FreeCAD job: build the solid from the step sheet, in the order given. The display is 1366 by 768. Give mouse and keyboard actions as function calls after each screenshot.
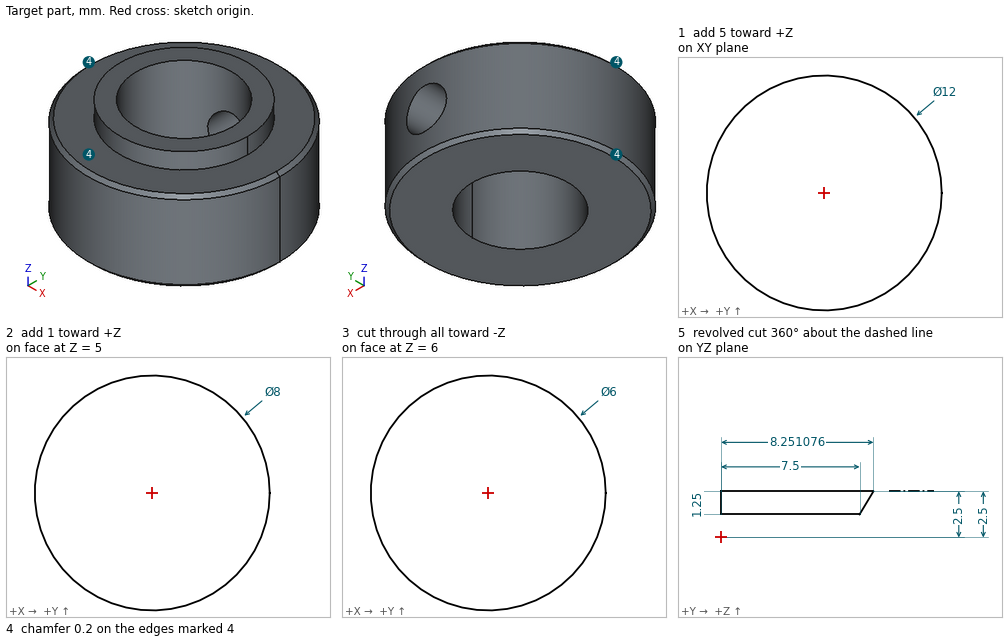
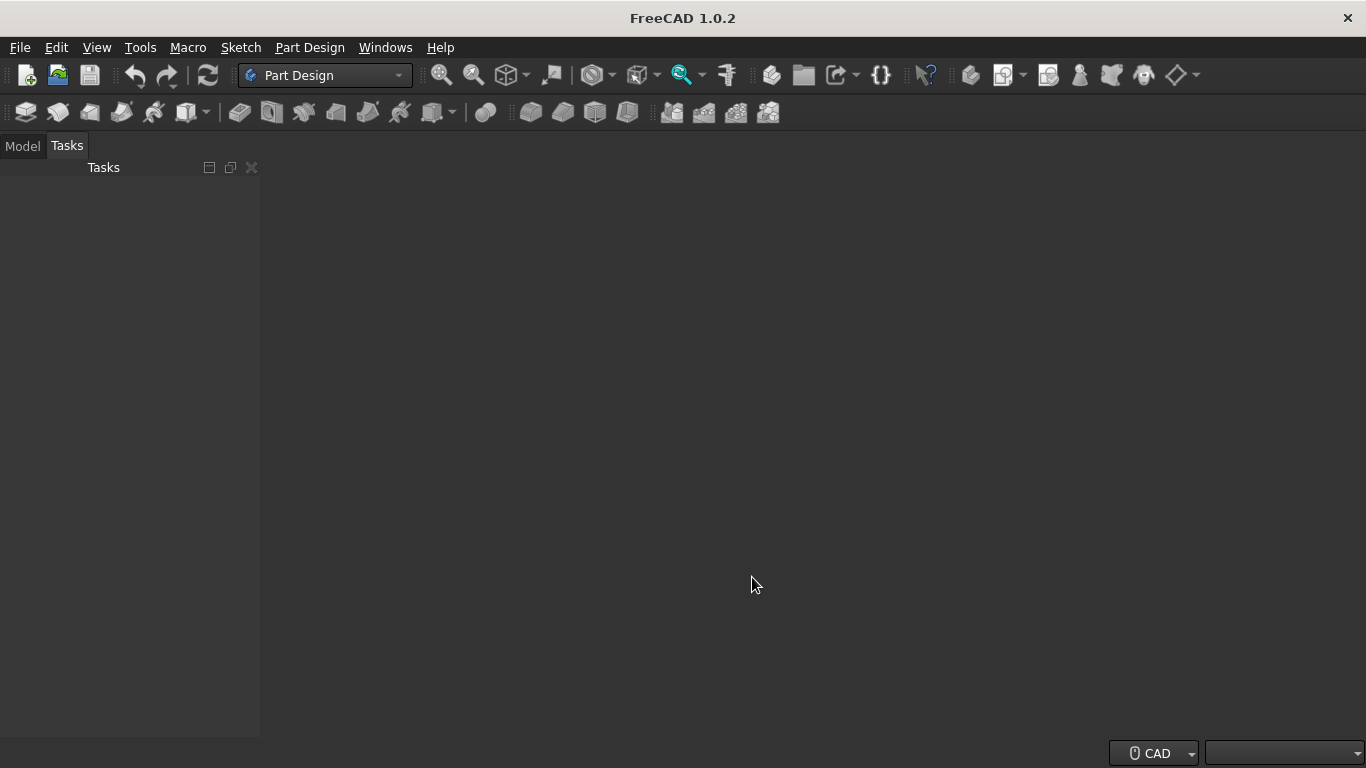
key(ctrl+n)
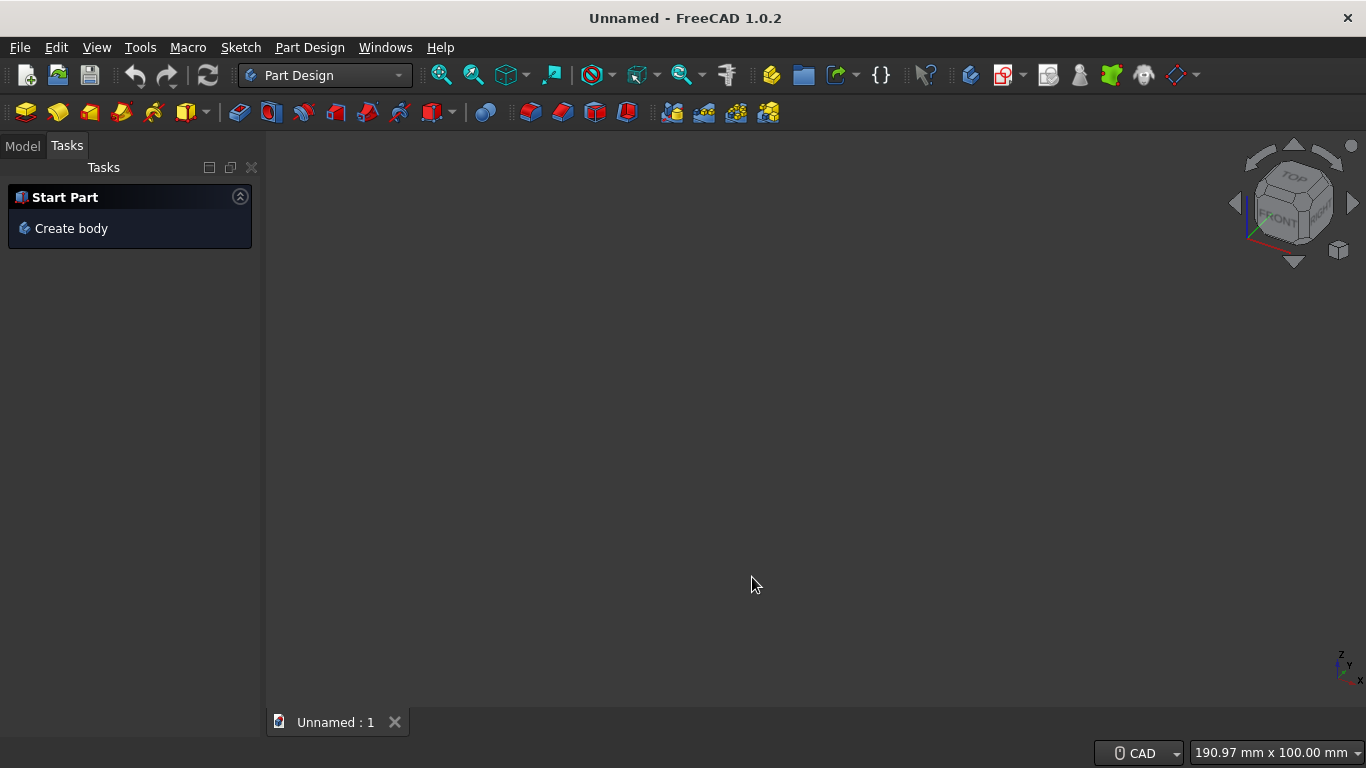
click(1004, 76)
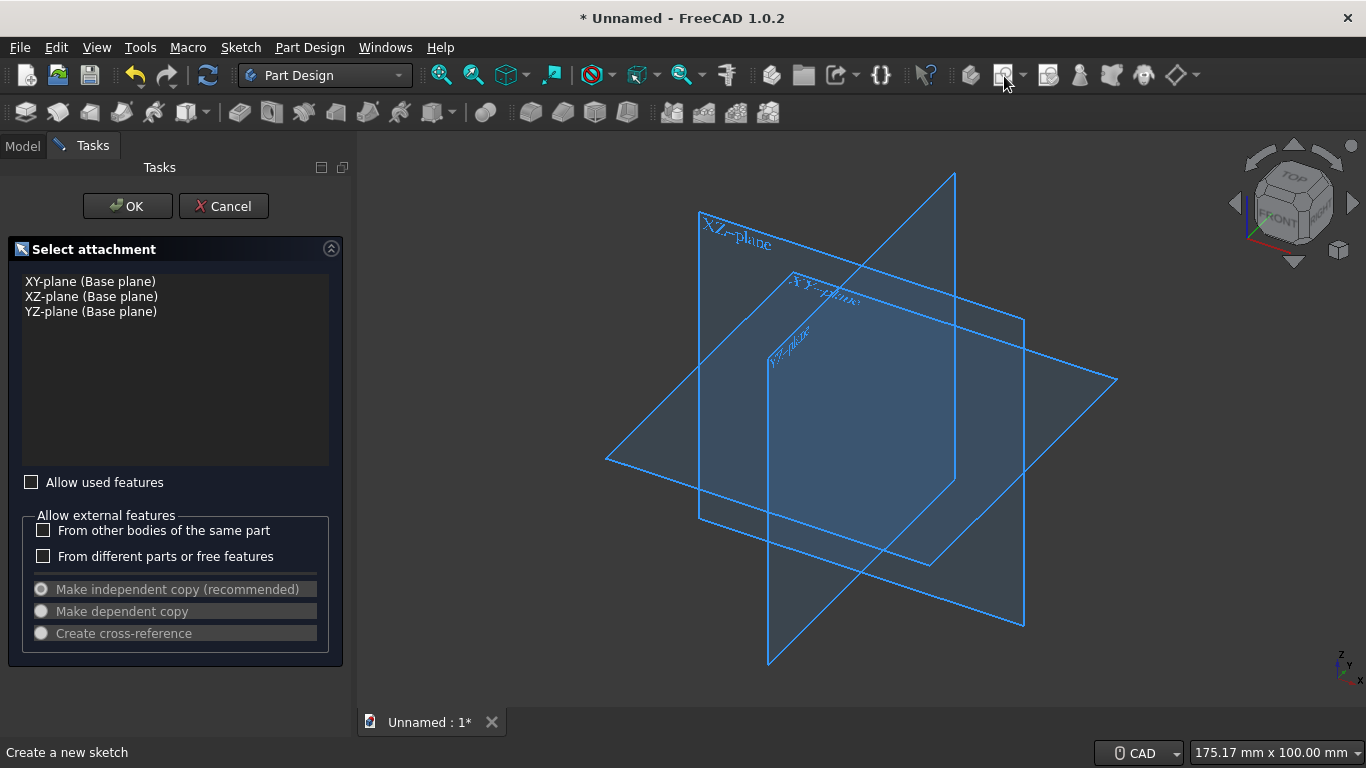
click(82, 282)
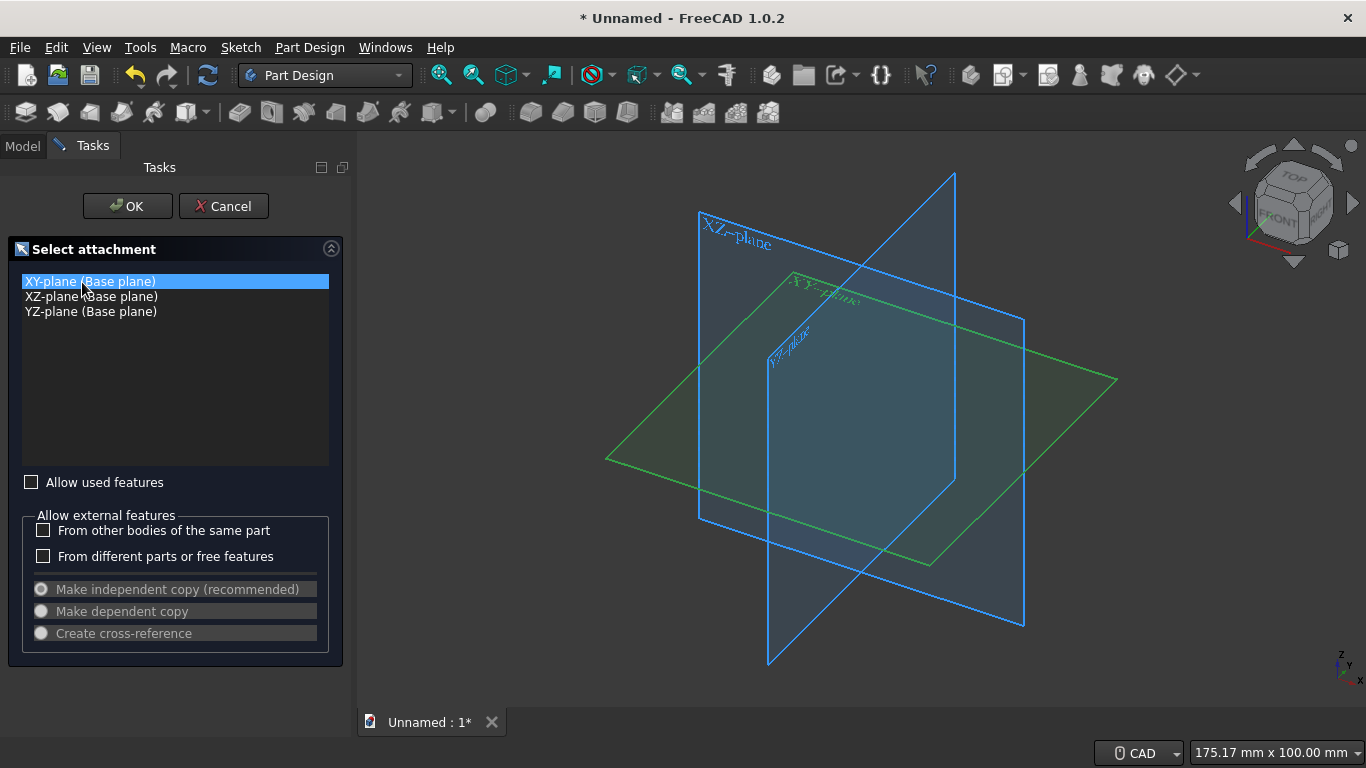
click(128, 206)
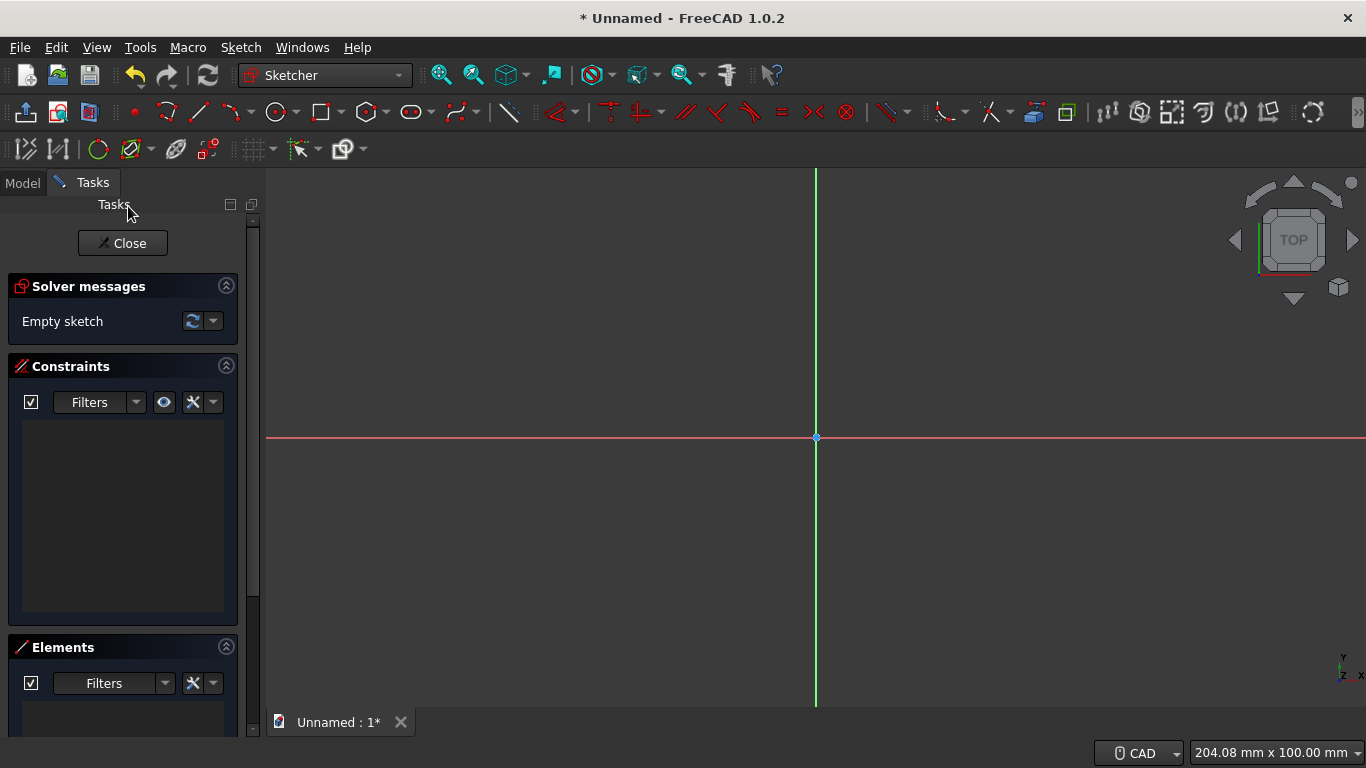
scroll(833, 438, up, 8)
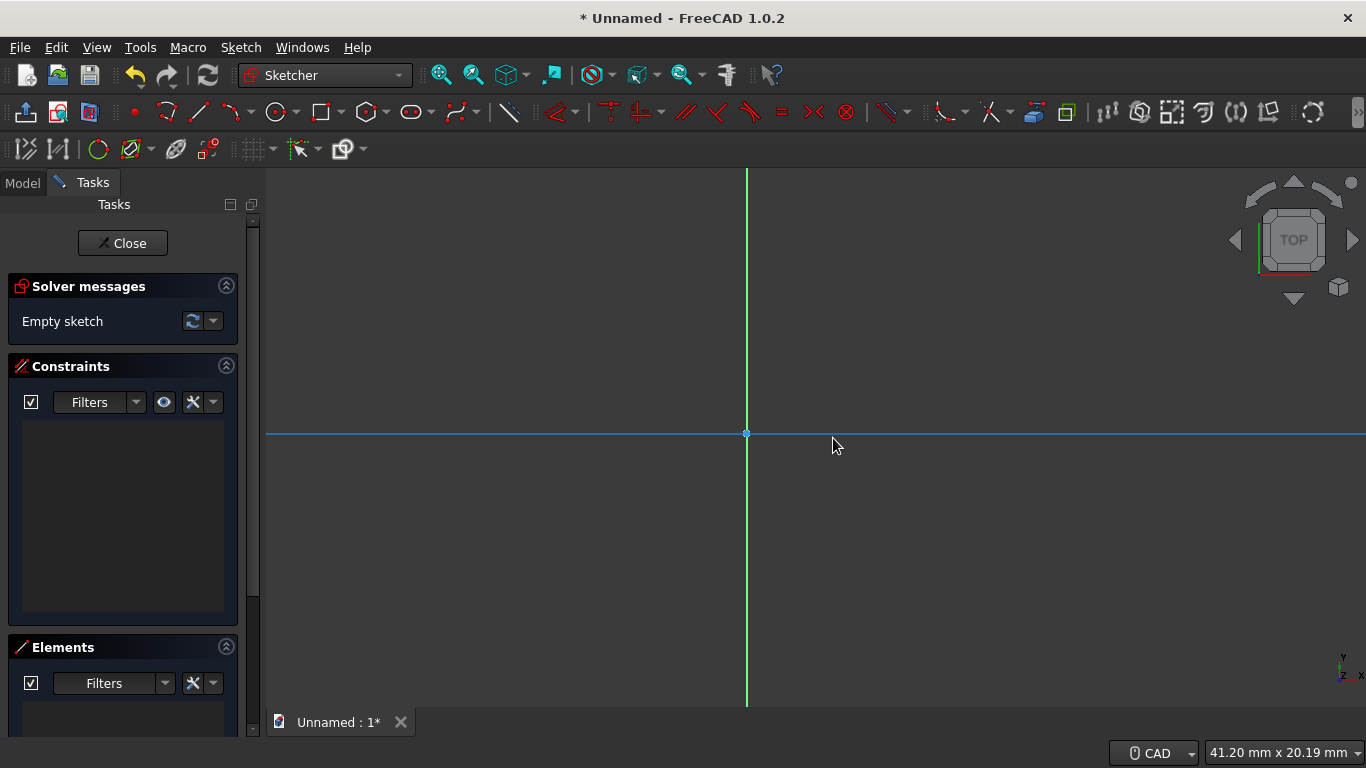
click(276, 112)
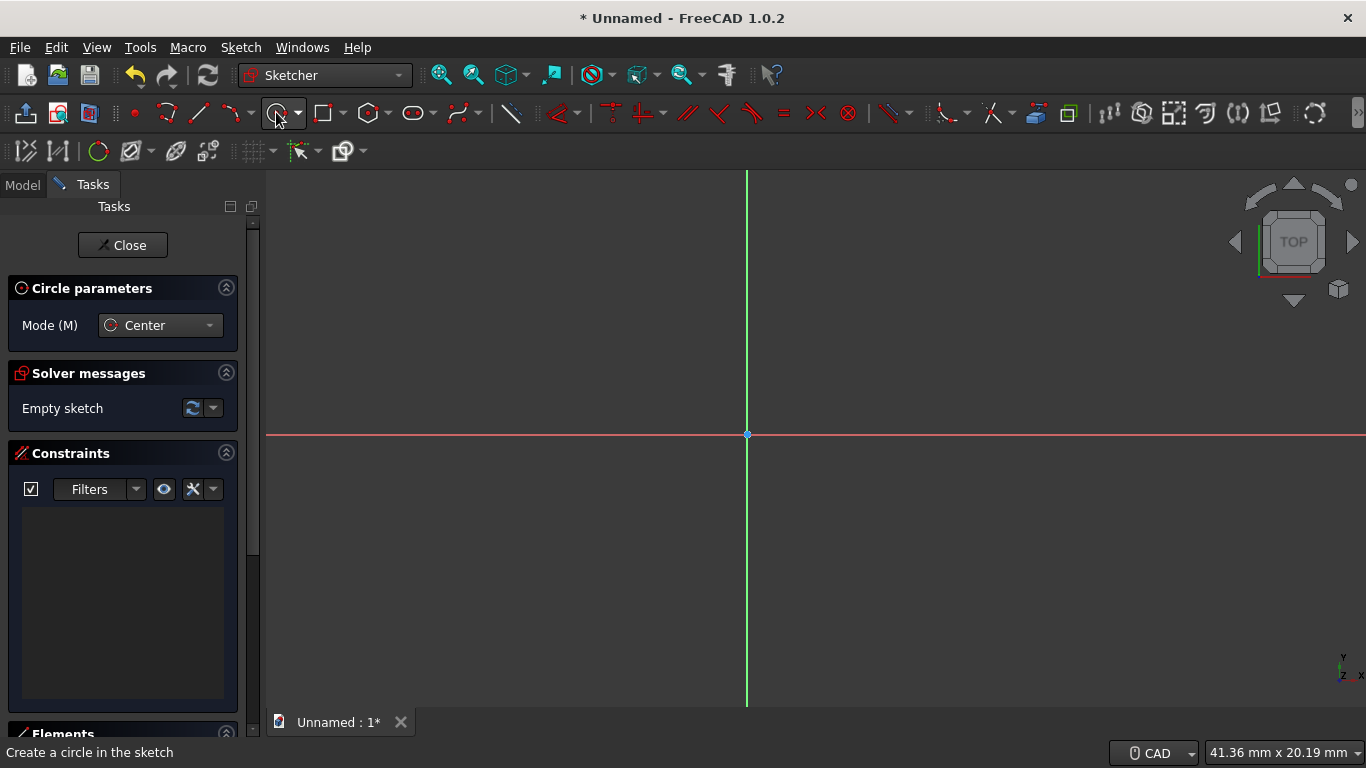
click(747, 435)
move(860, 322)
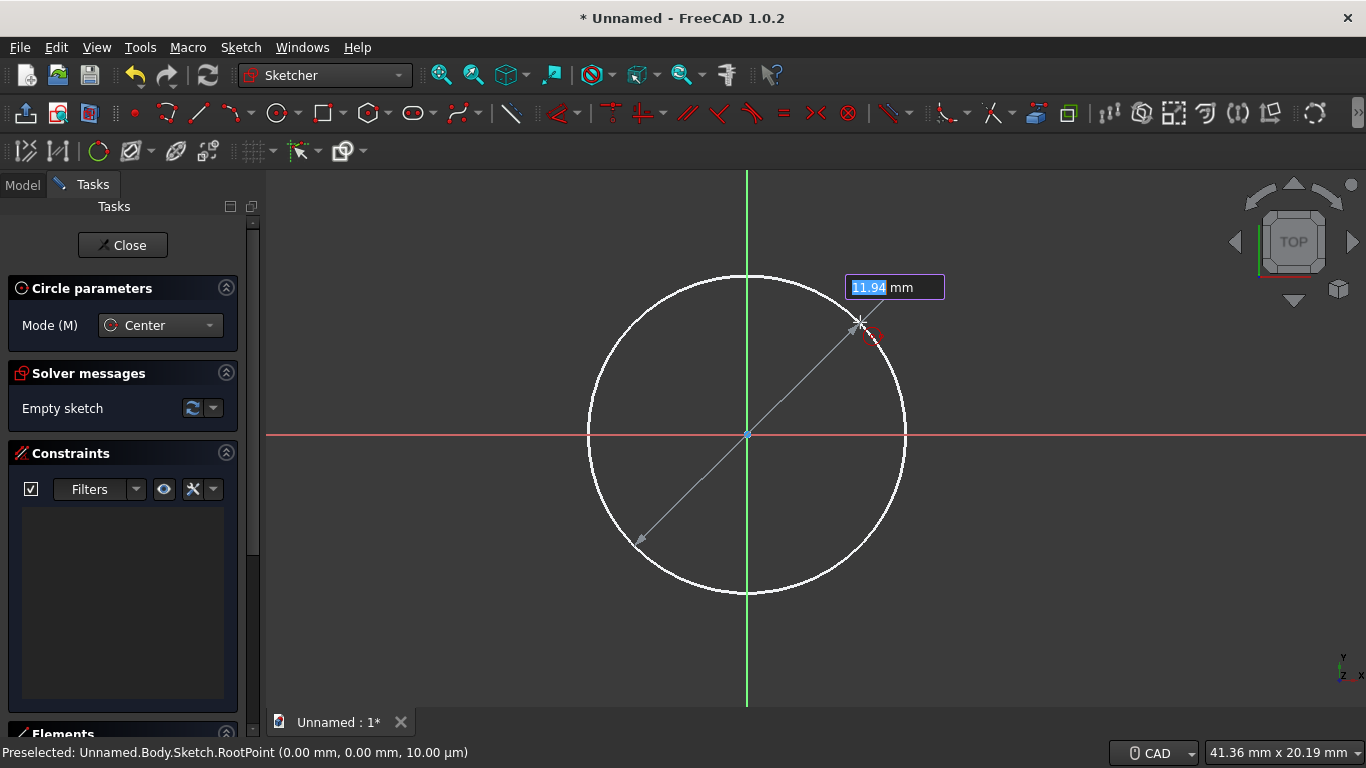
text(12)
key(Return)
key(Escape)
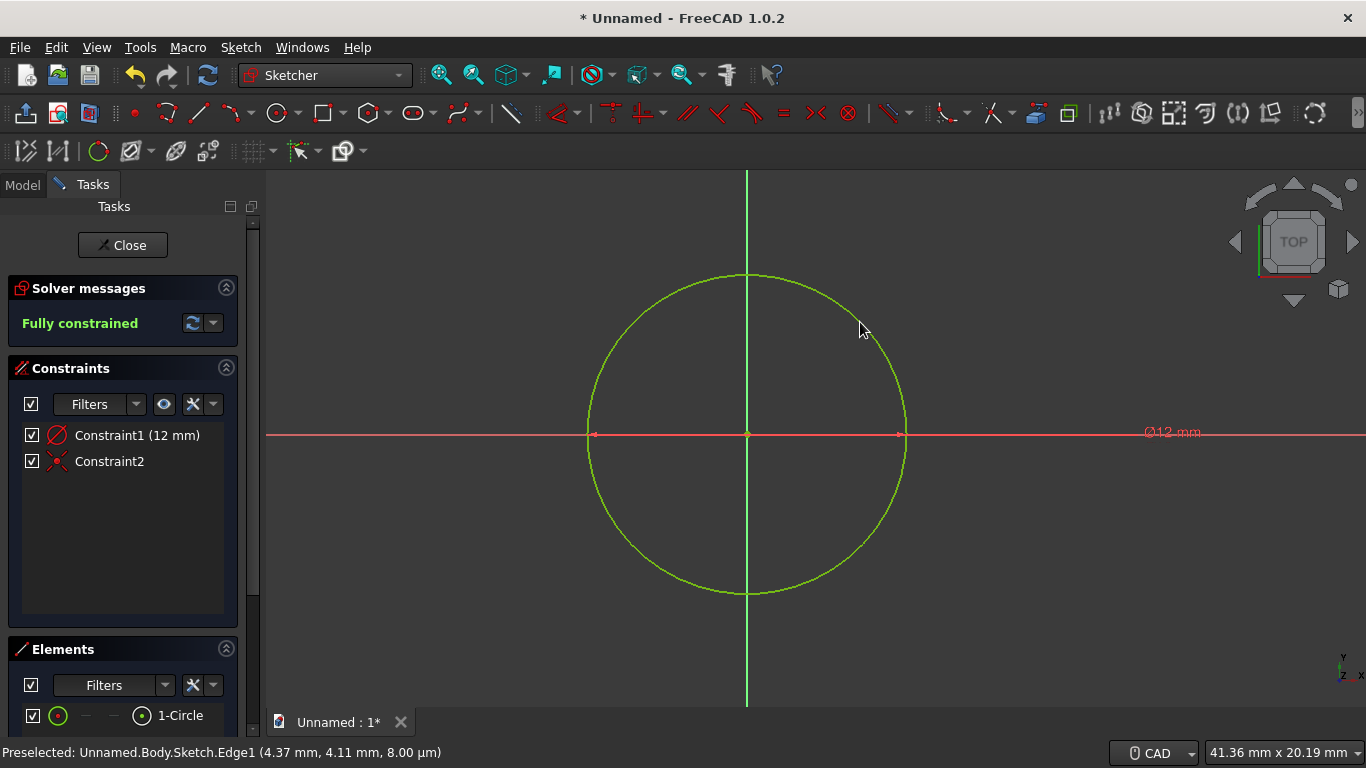
click(123, 245)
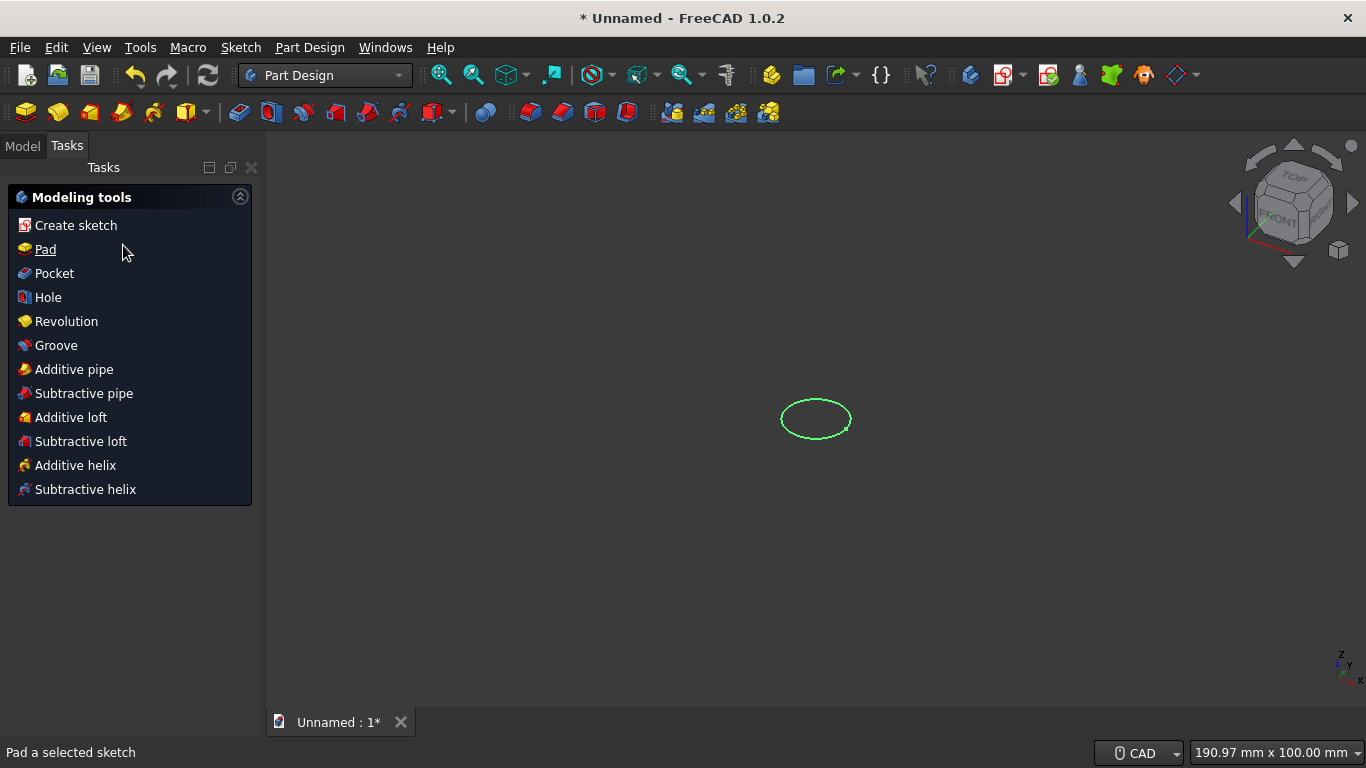
click(26, 112)